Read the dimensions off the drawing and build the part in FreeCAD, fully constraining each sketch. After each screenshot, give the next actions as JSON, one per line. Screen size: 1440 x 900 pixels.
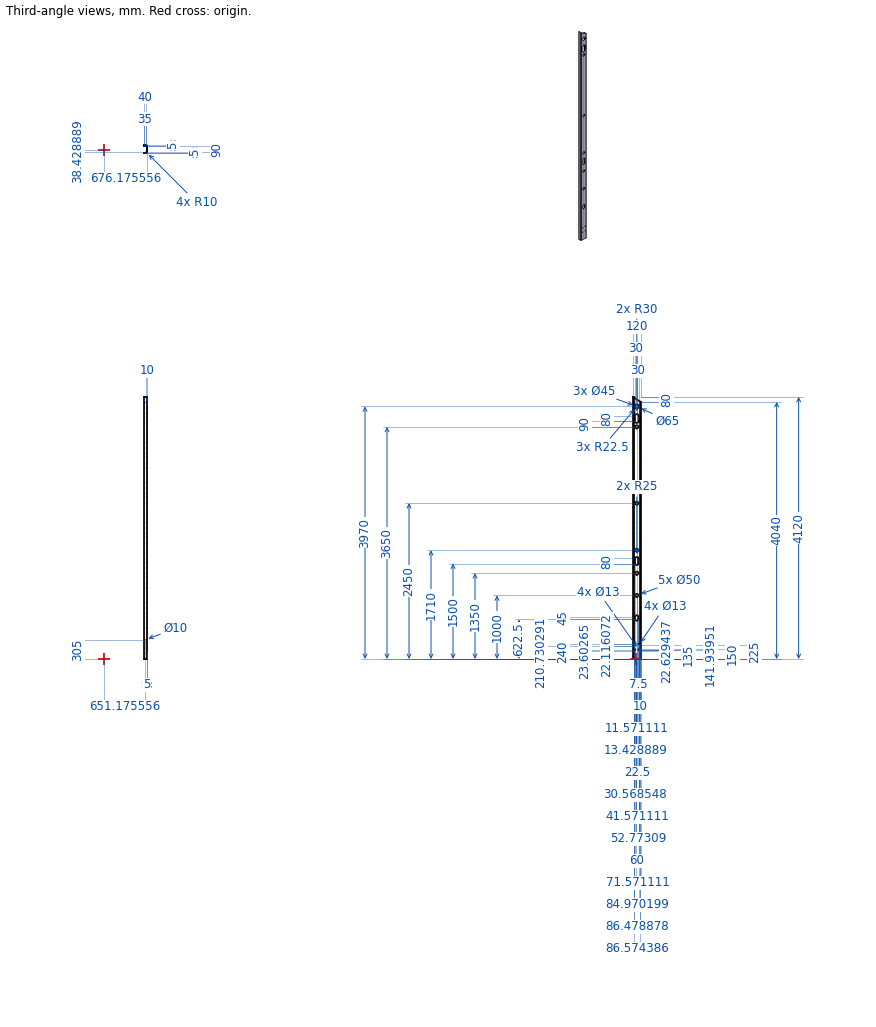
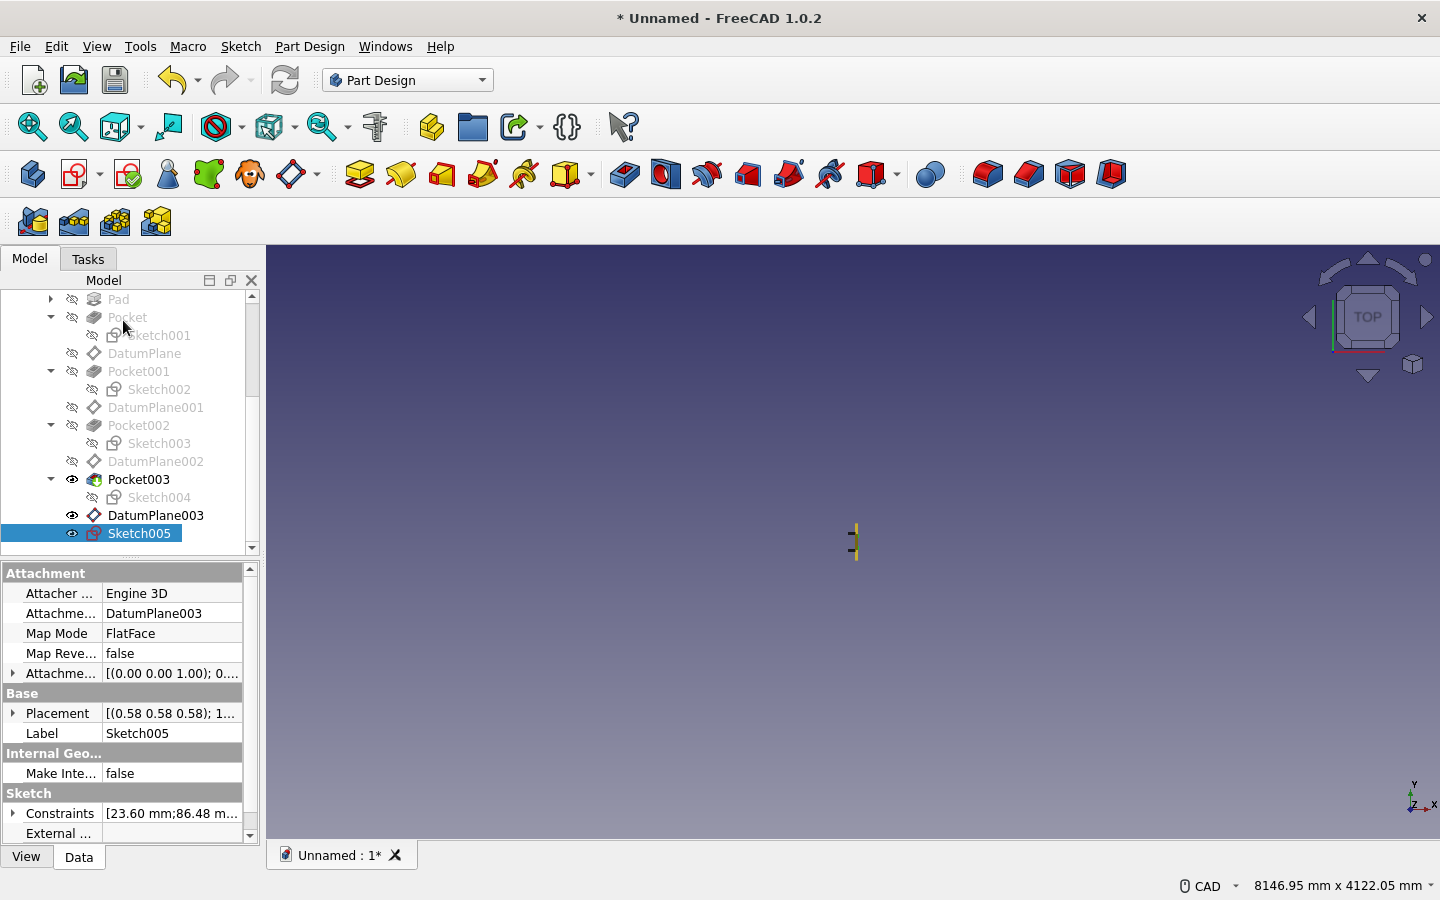
{"action": "left_click", "coordinate": [360, 174]}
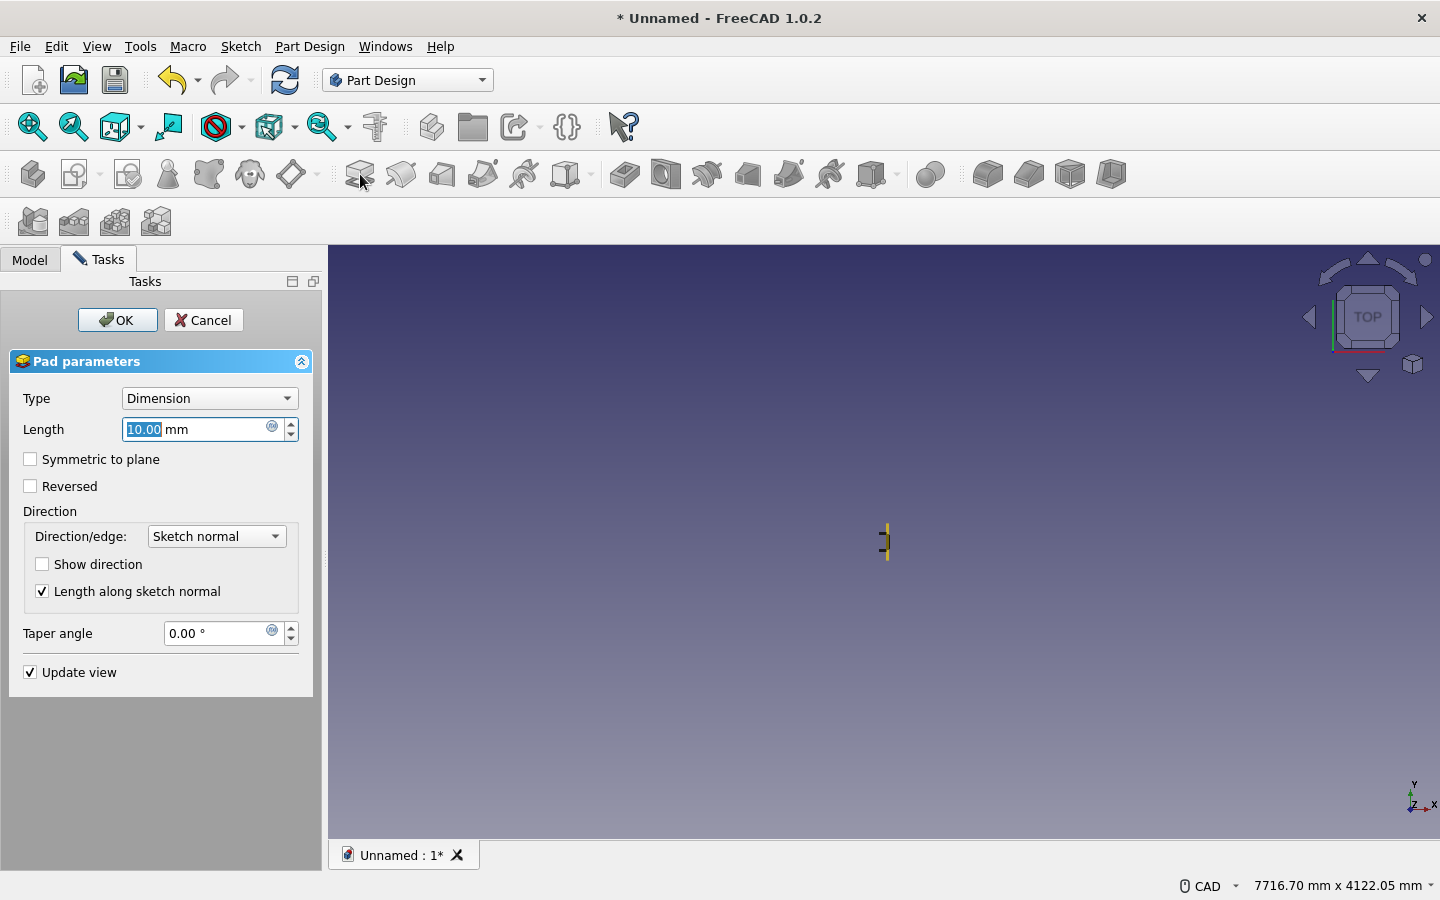
{"action": "type", "text": "5"}
{"action": "key", "text": "Tab"}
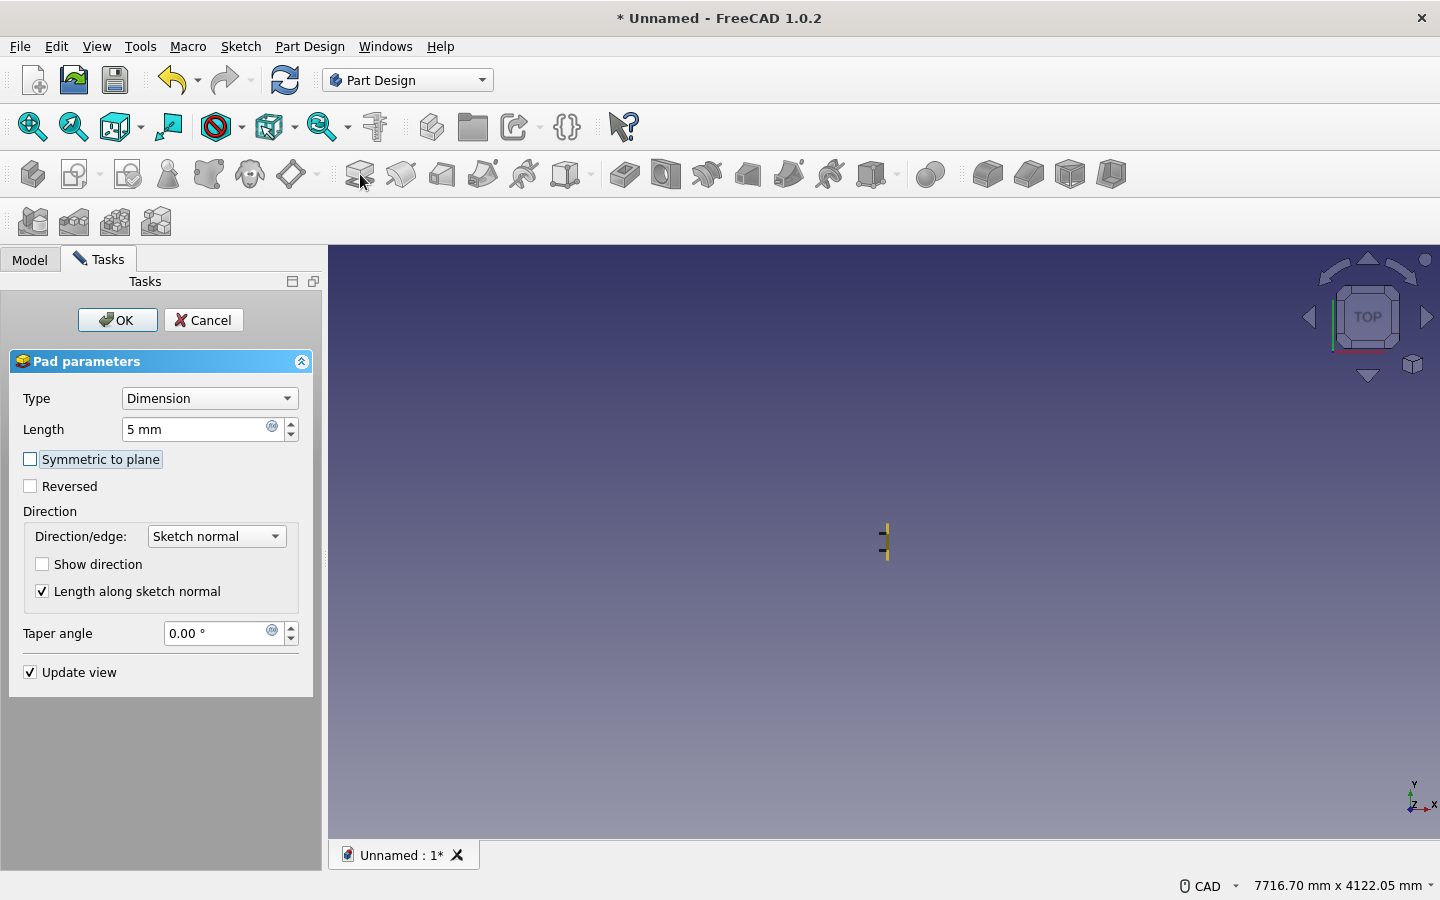
{"action": "left_click", "coordinate": [31, 486]}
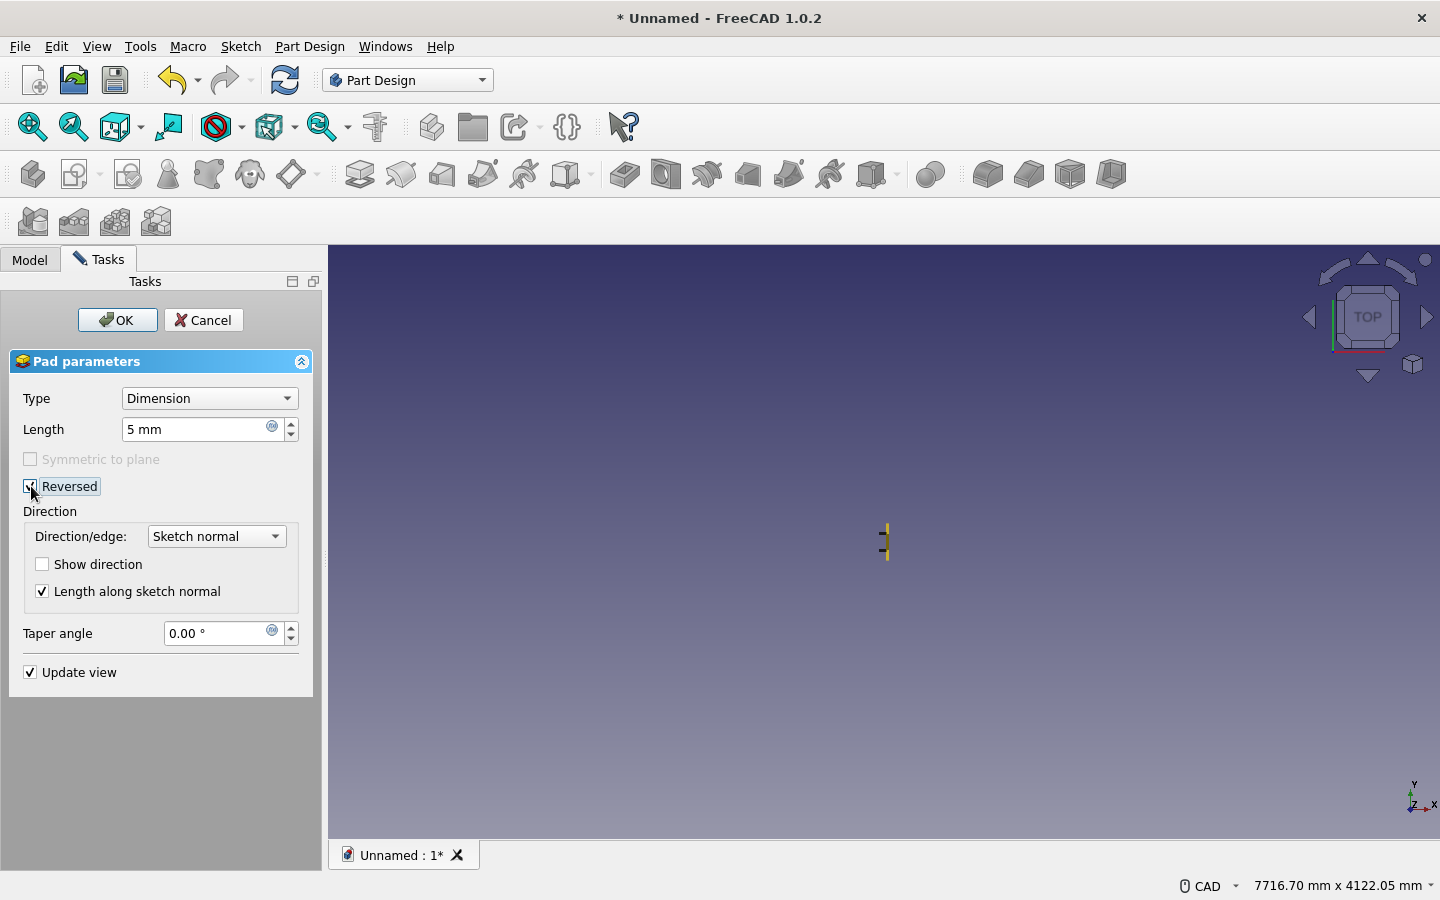
{"action": "left_click", "coordinate": [118, 320]}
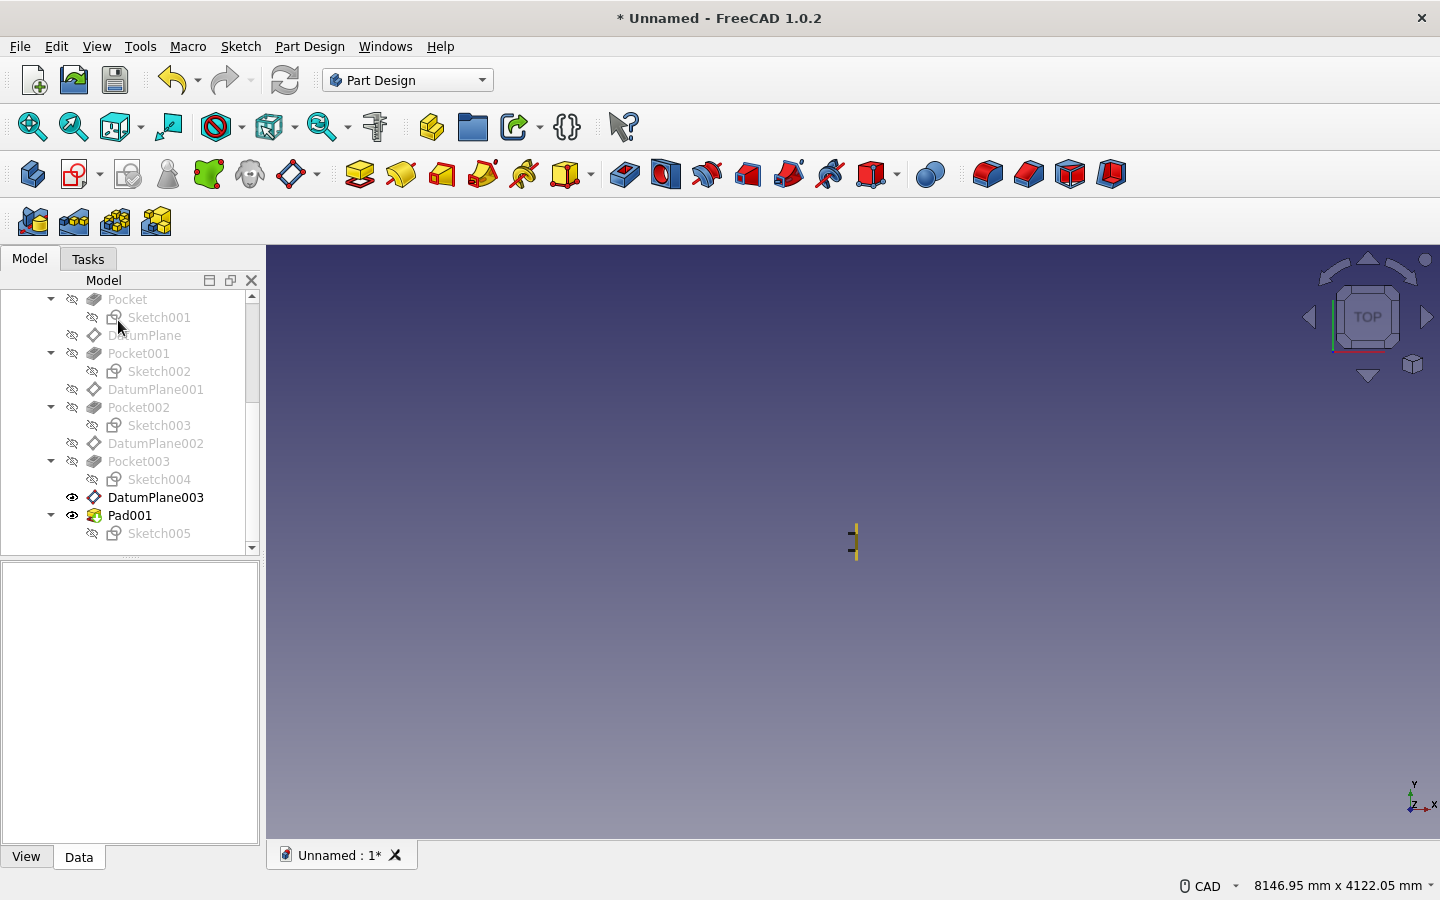
{"action": "left_click", "coordinate": [117, 497]}
{"action": "key", "text": "space"}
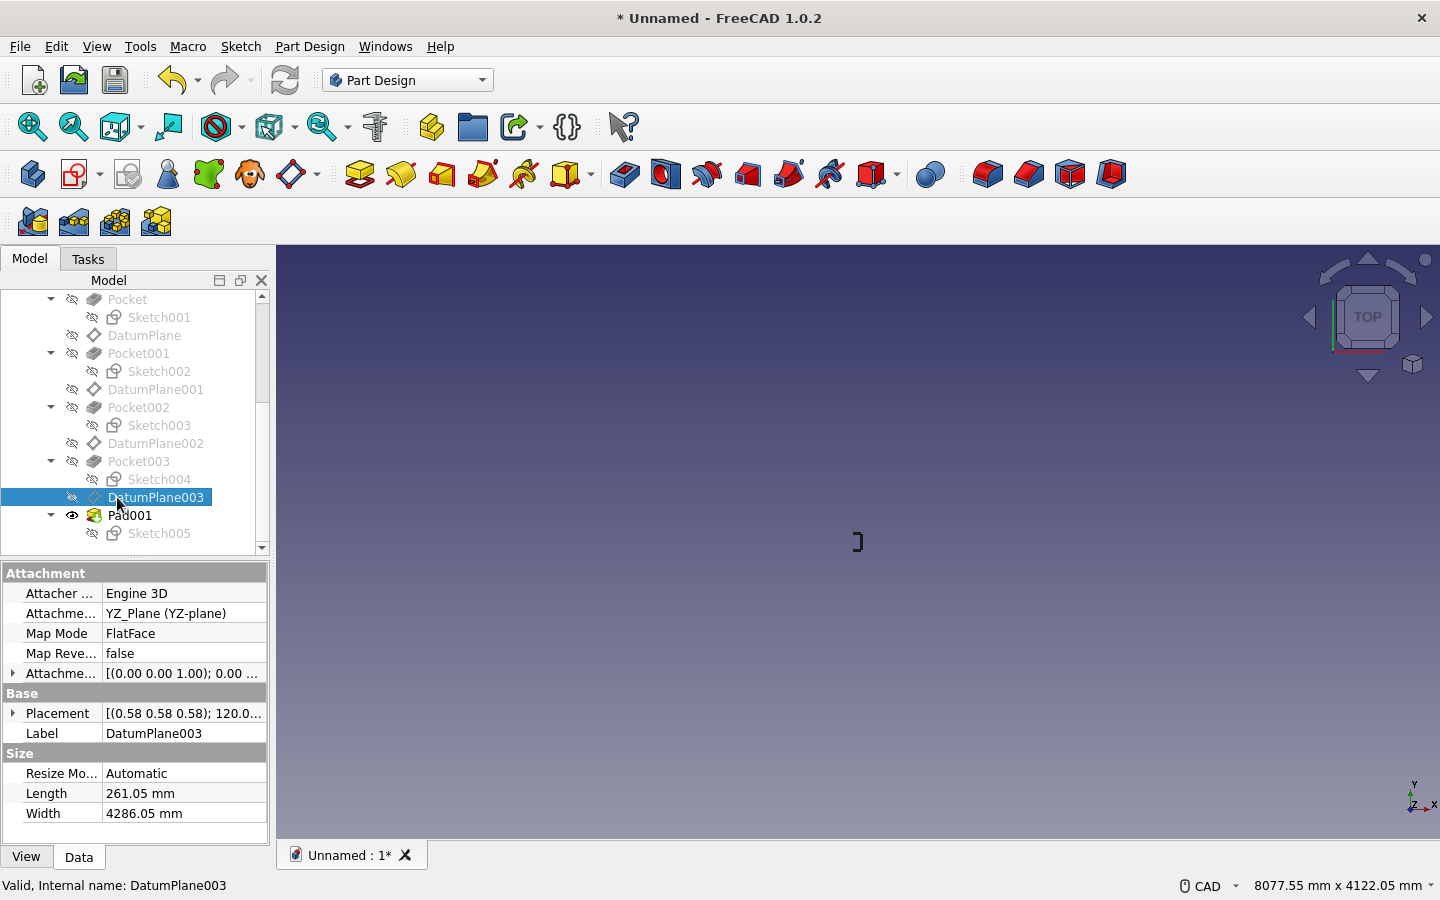
{"action": "left_click", "coordinate": [33, 128]}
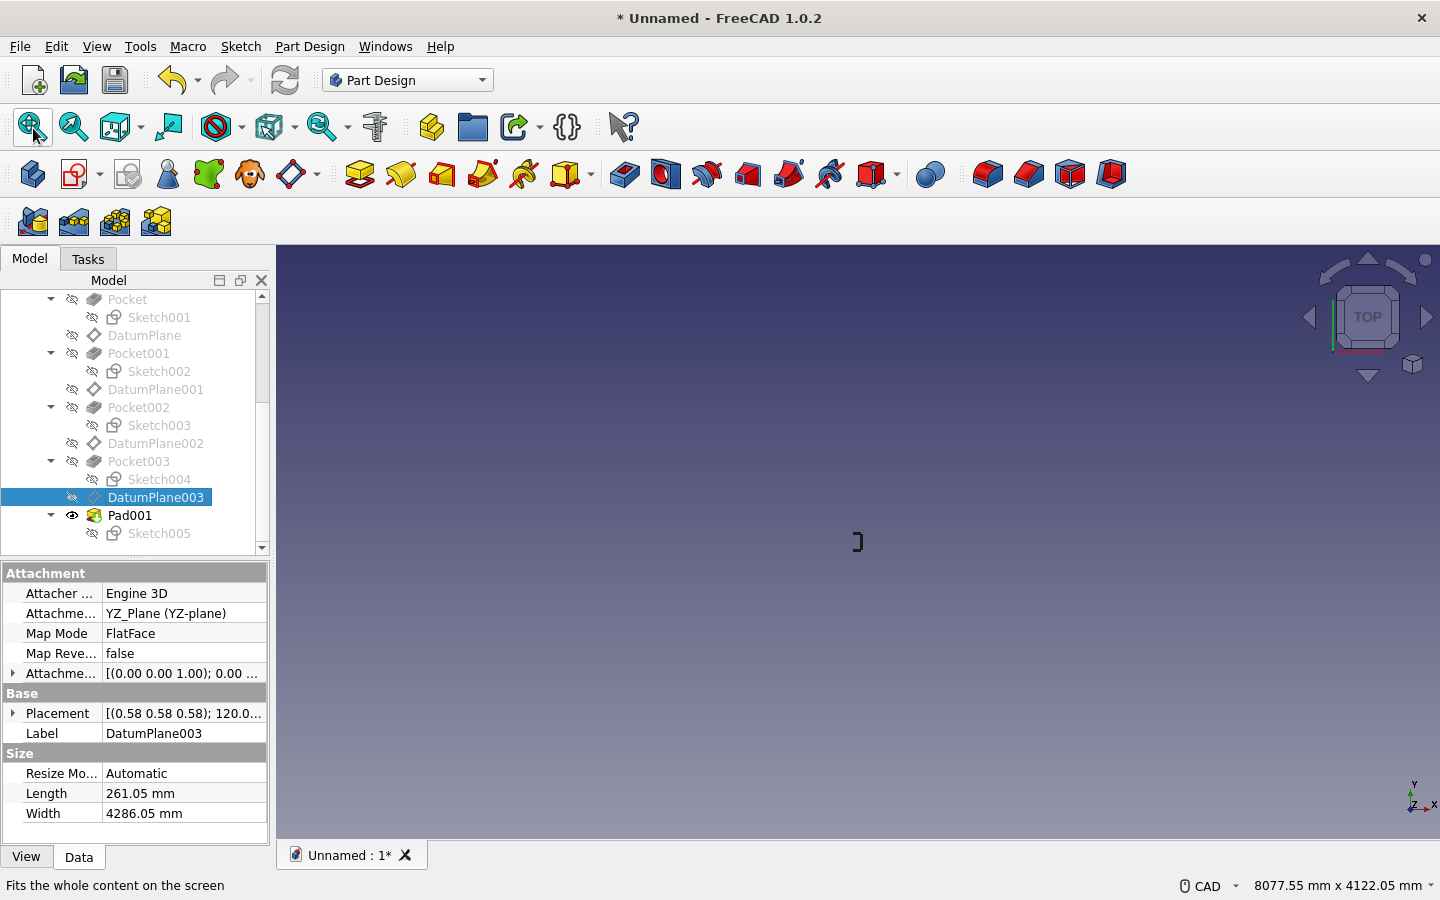
{"action": "key", "text": "0"}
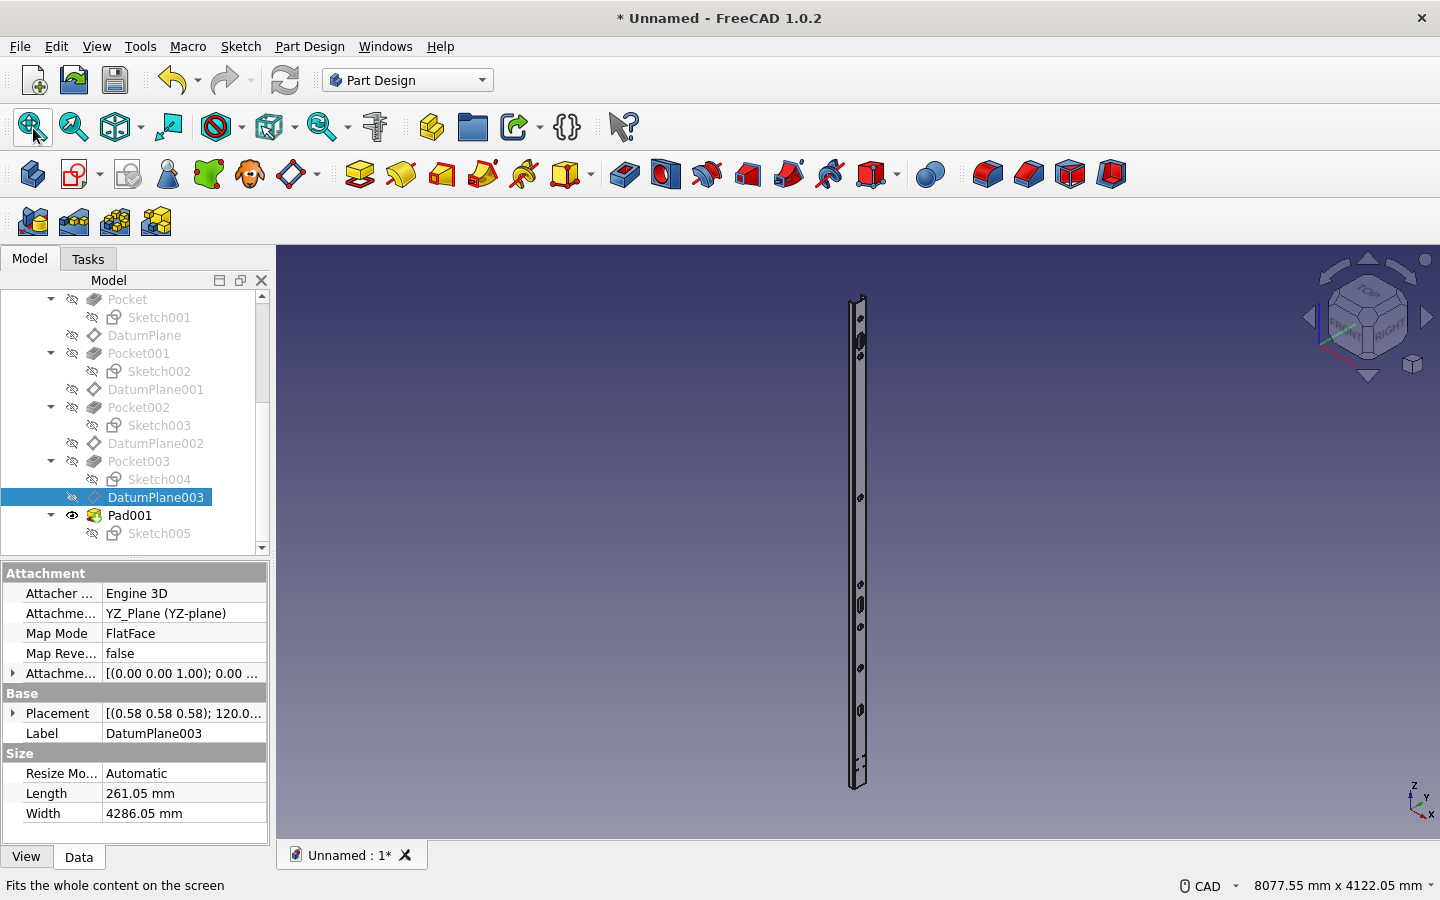
{"action": "key", "text": "3"}